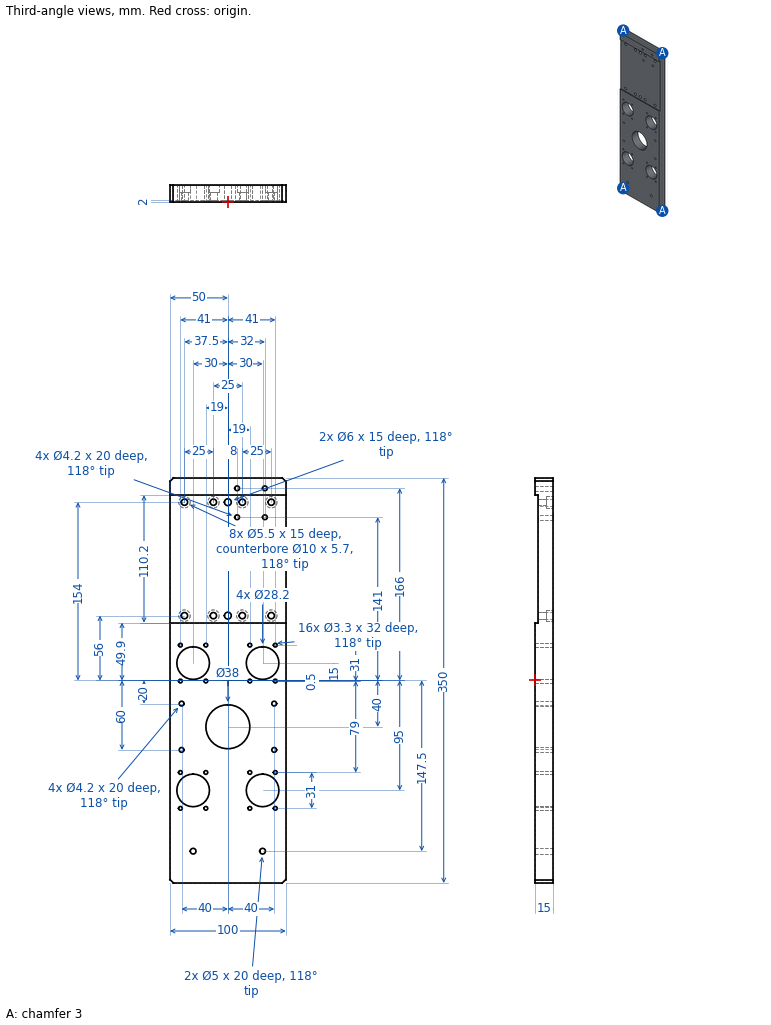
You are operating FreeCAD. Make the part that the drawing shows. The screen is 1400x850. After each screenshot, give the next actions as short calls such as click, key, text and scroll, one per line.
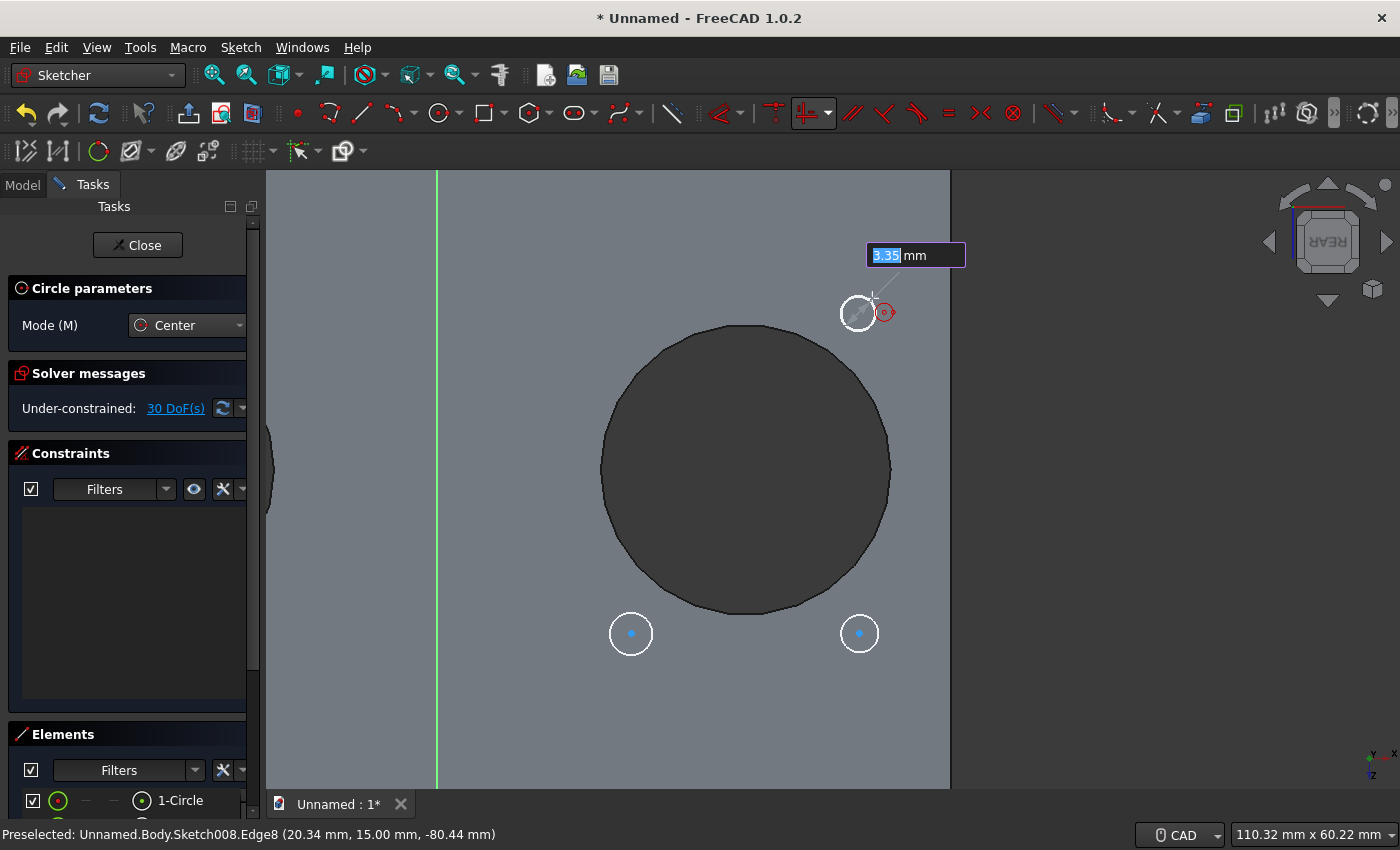
click(871, 299)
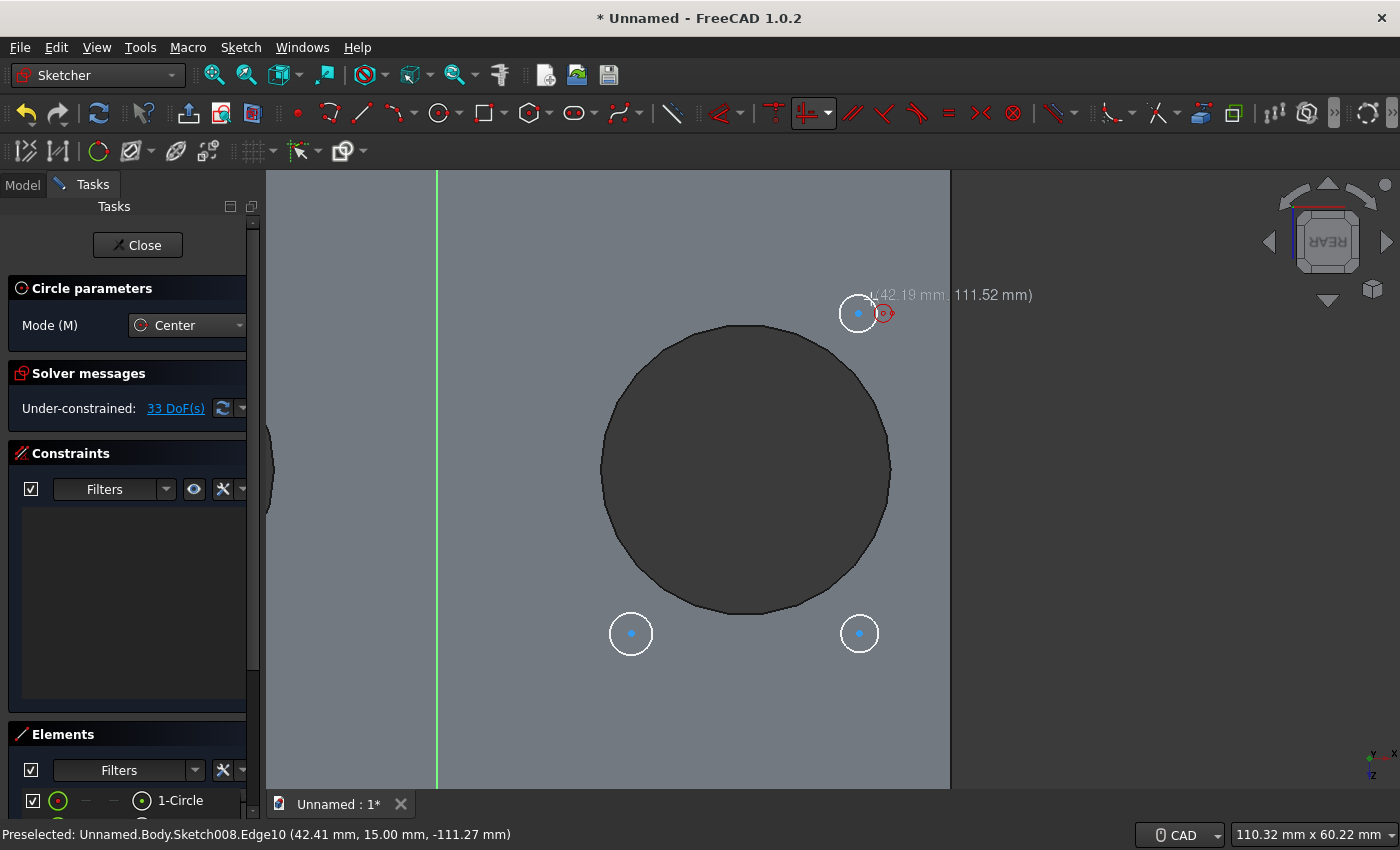
scroll(633, 311, up, 2)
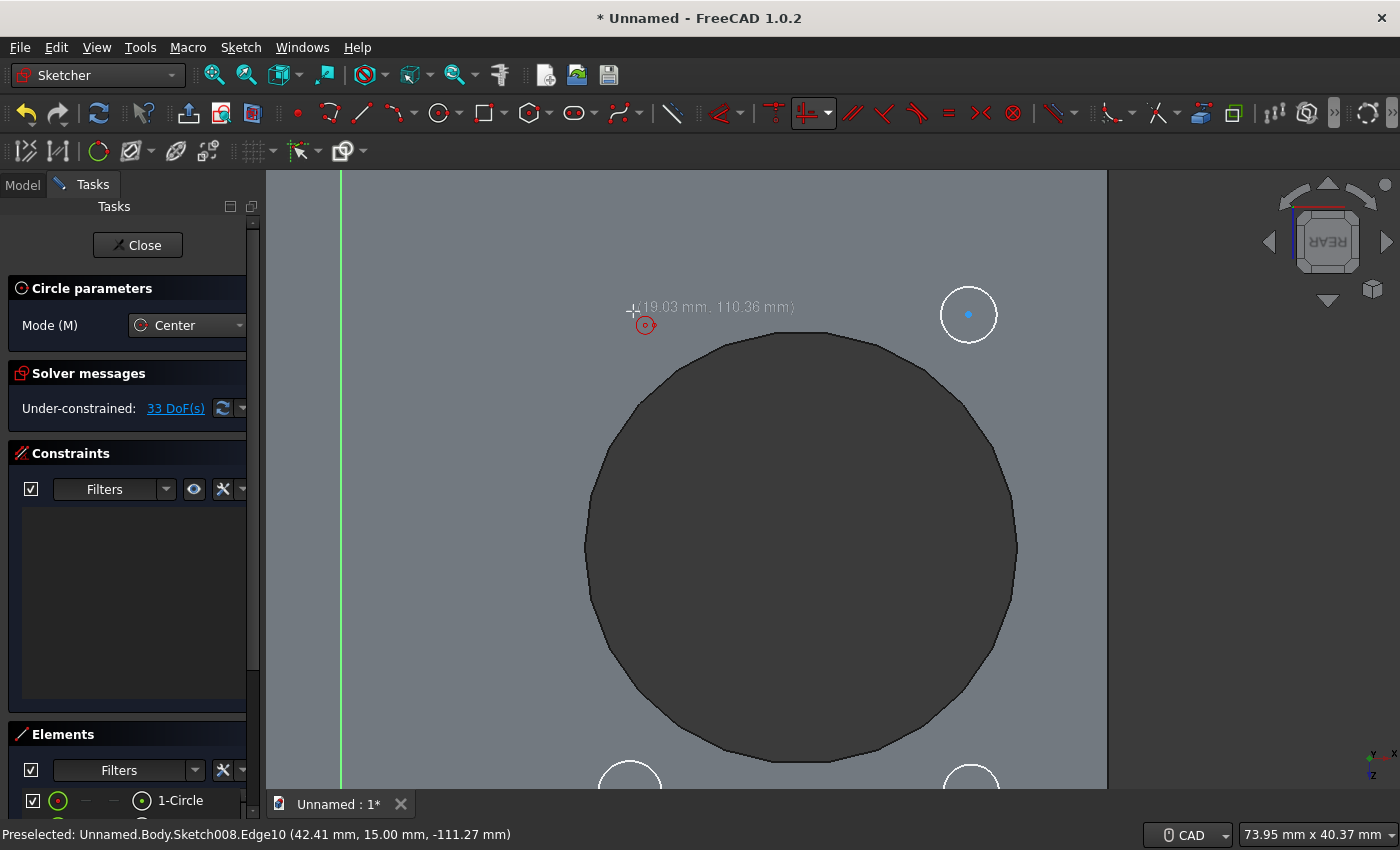
scroll(848, 299, down, 9)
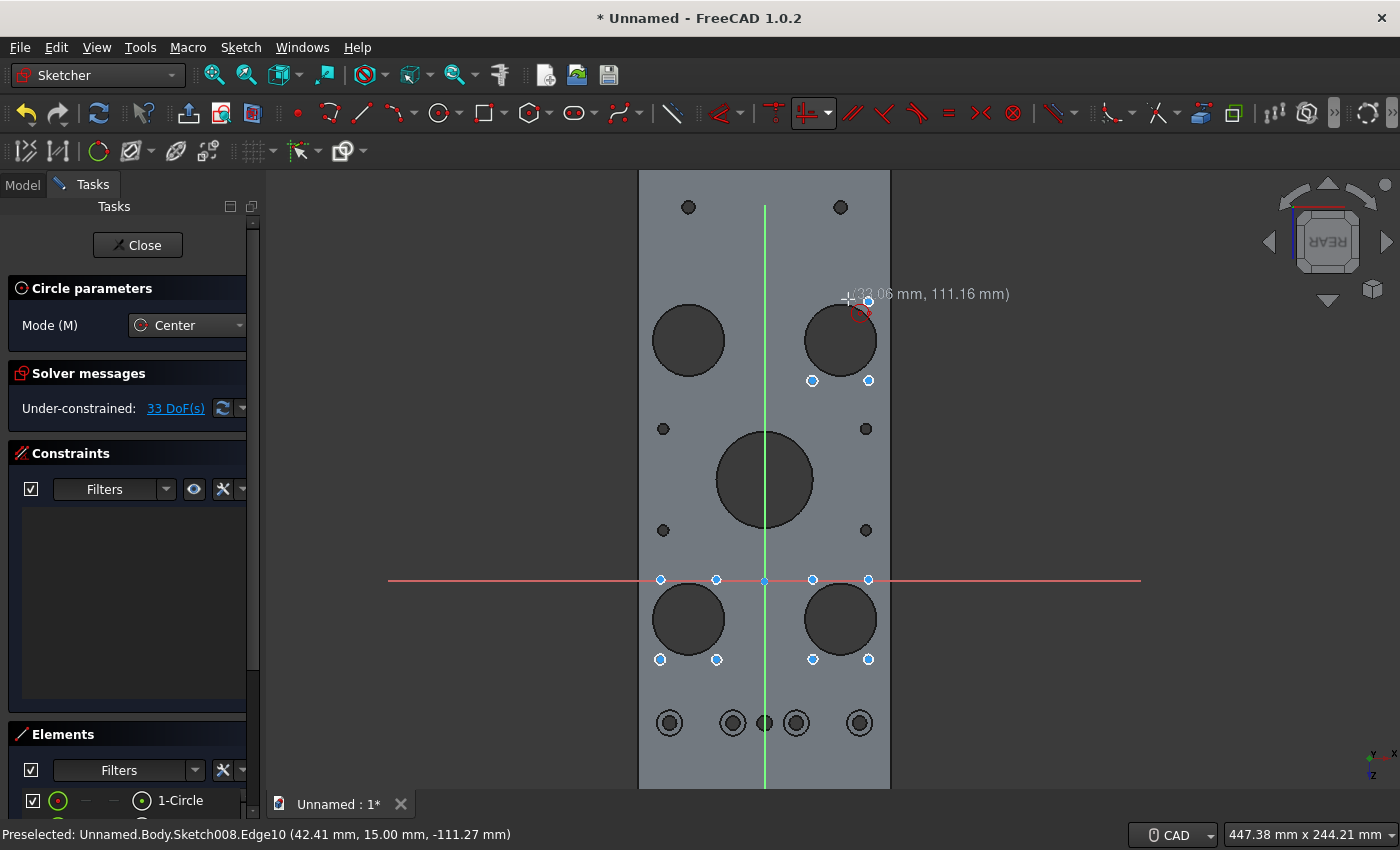
click(813, 301)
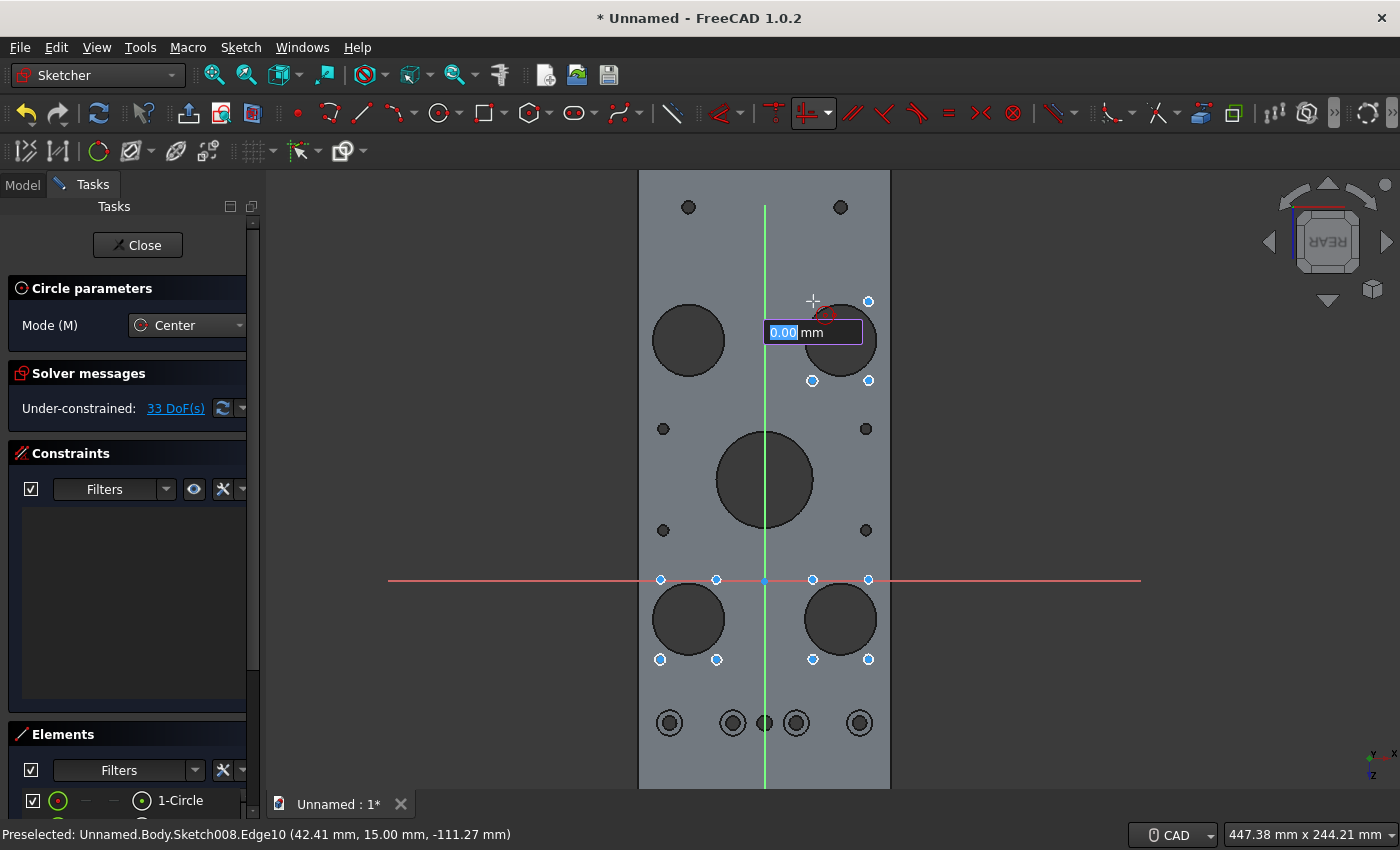
scroll(816, 298, up, 7)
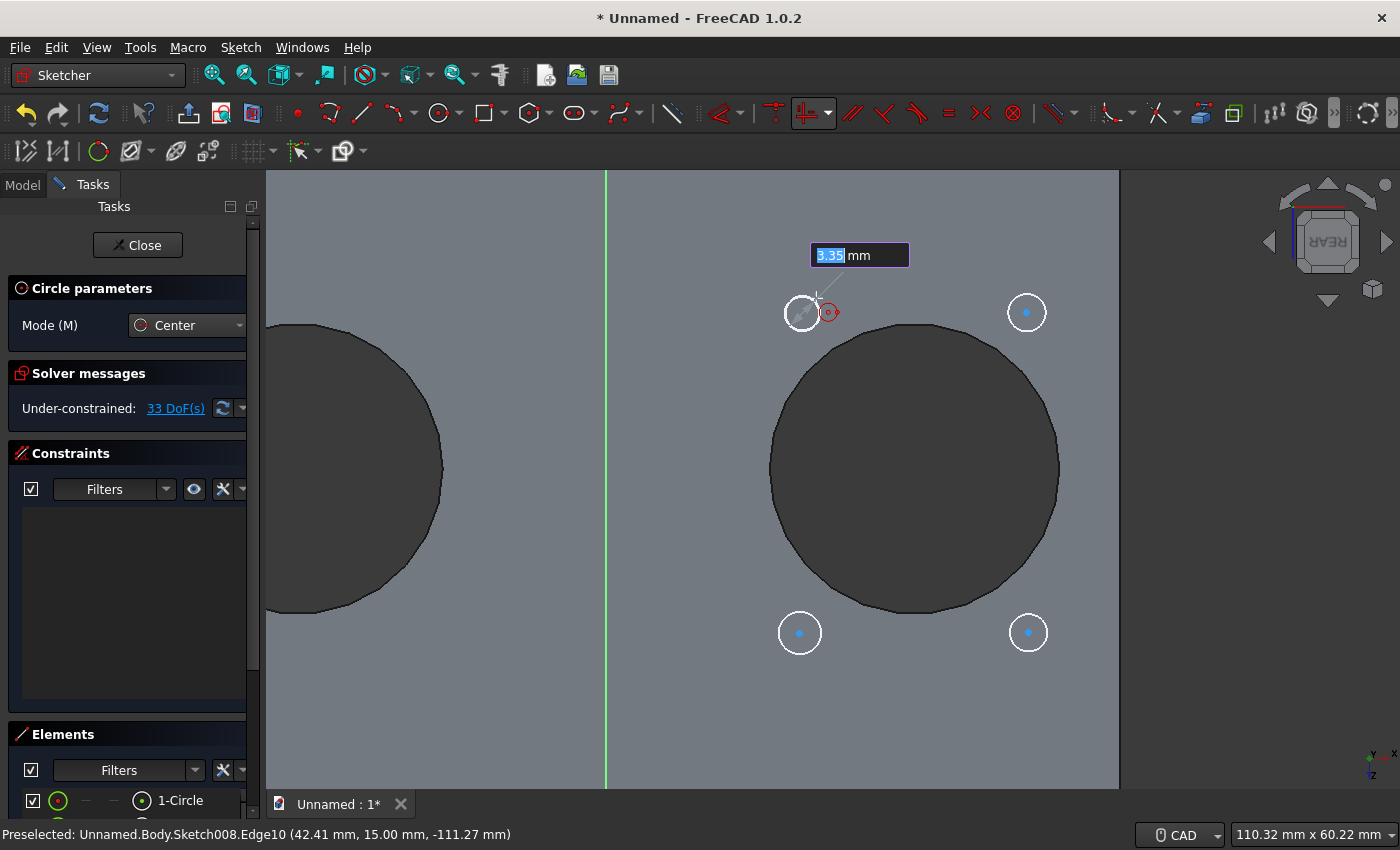
click(813, 298)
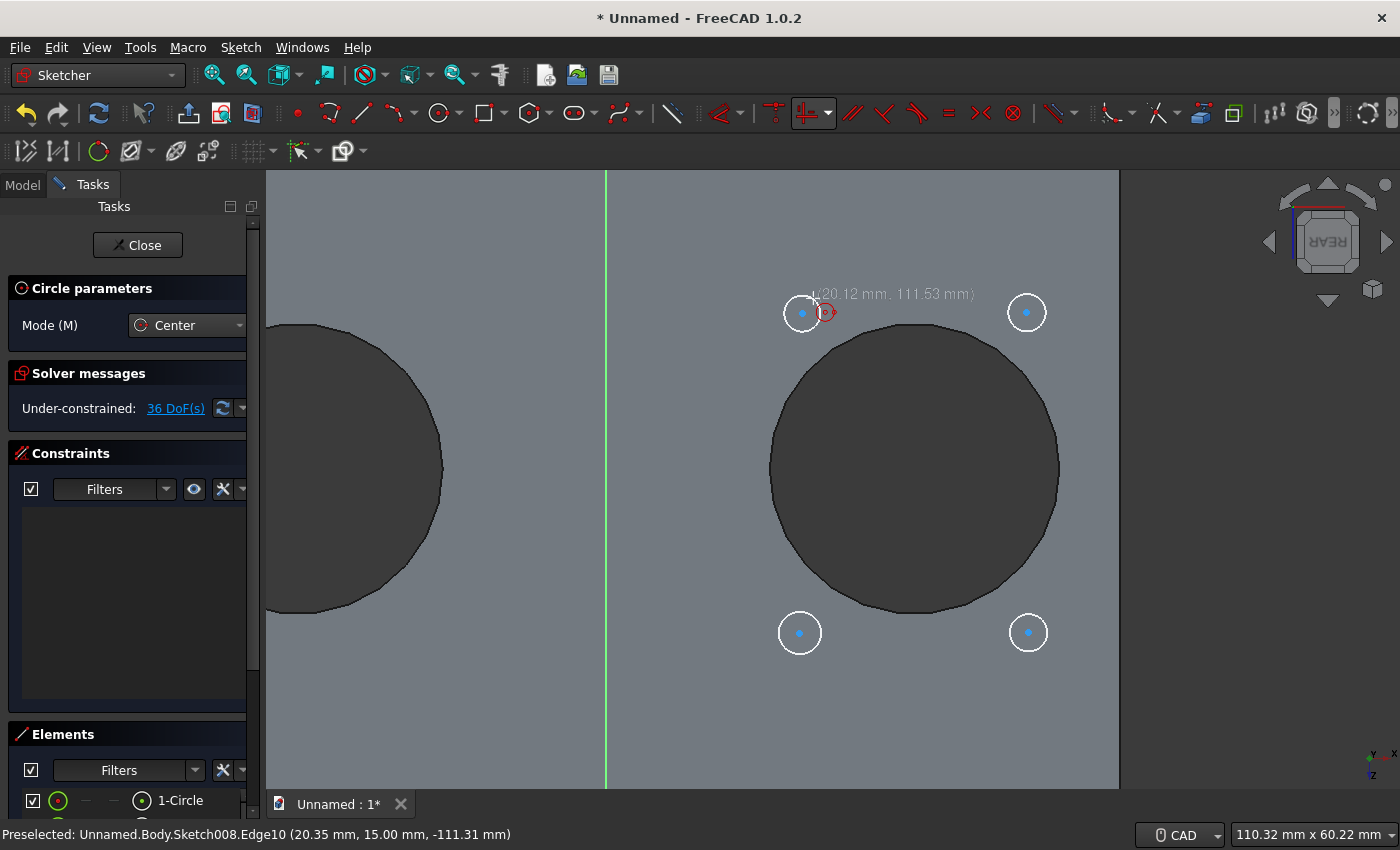
scroll(411, 628, up, 2)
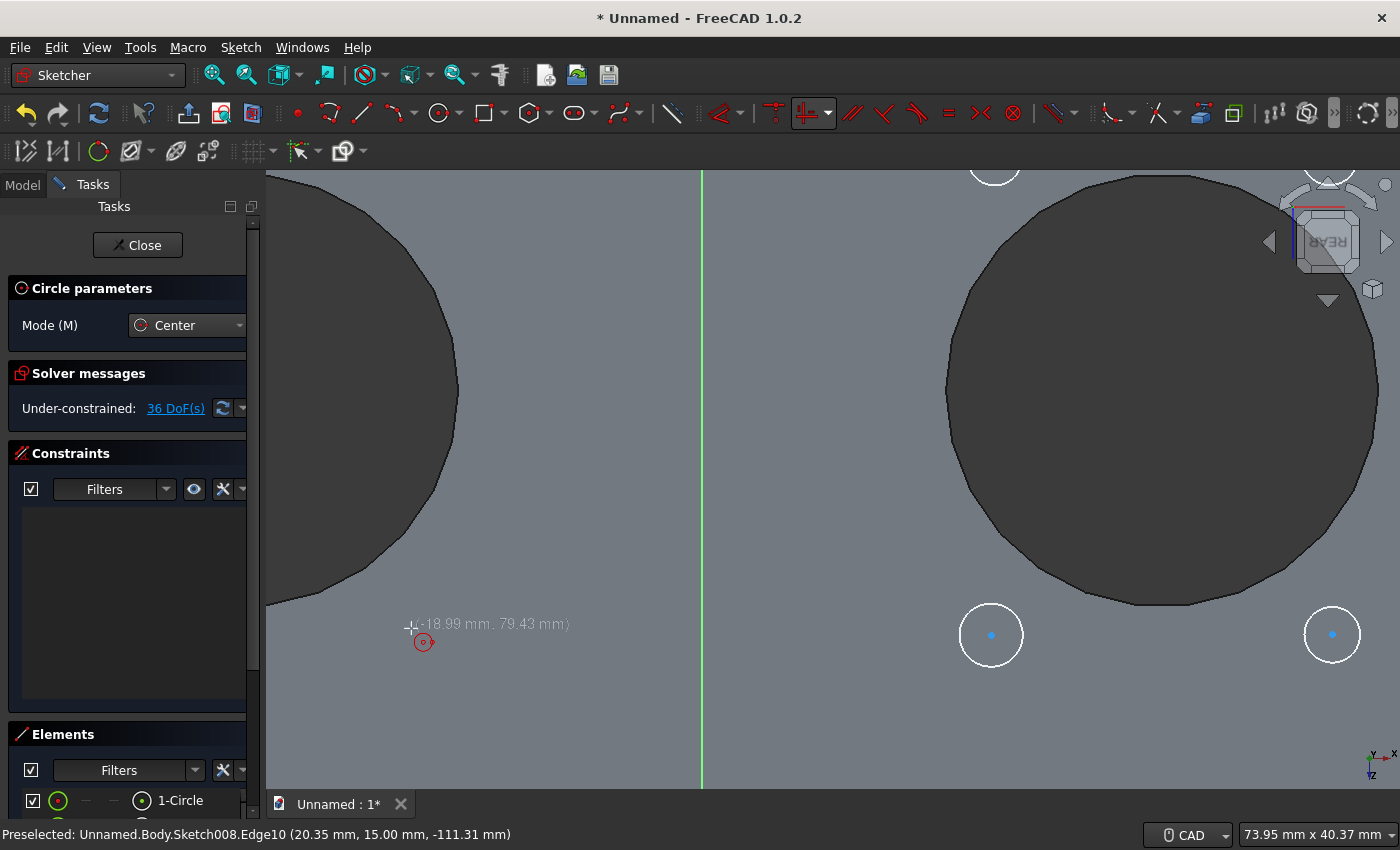
scroll(777, 330, down, 9)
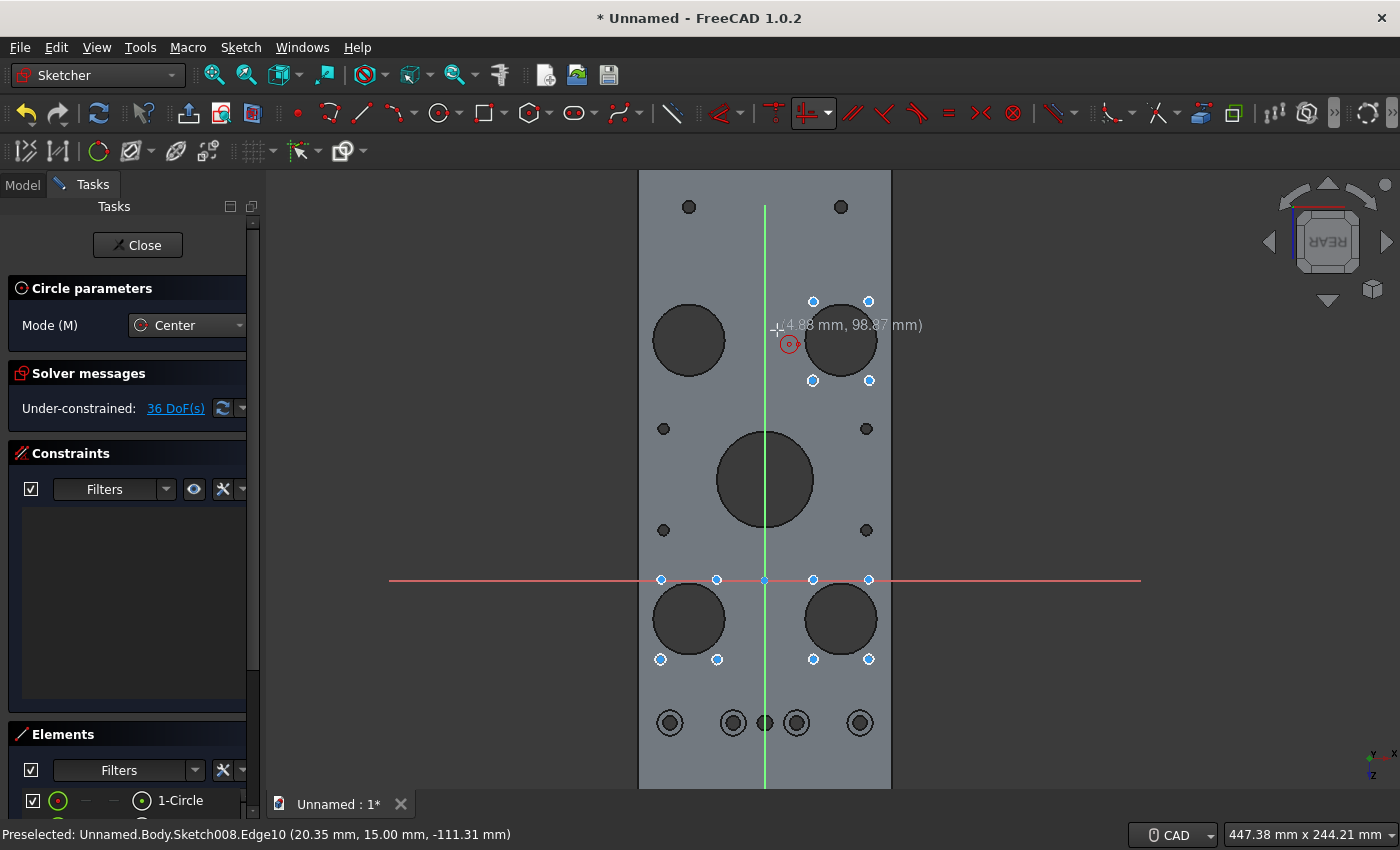
click(717, 379)